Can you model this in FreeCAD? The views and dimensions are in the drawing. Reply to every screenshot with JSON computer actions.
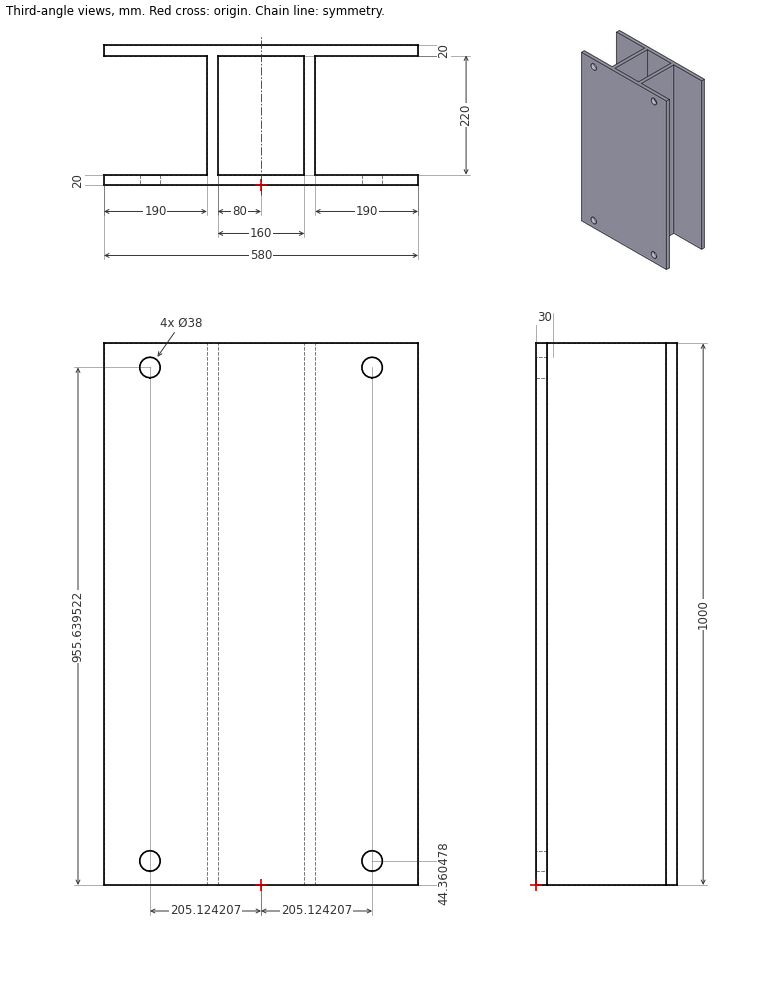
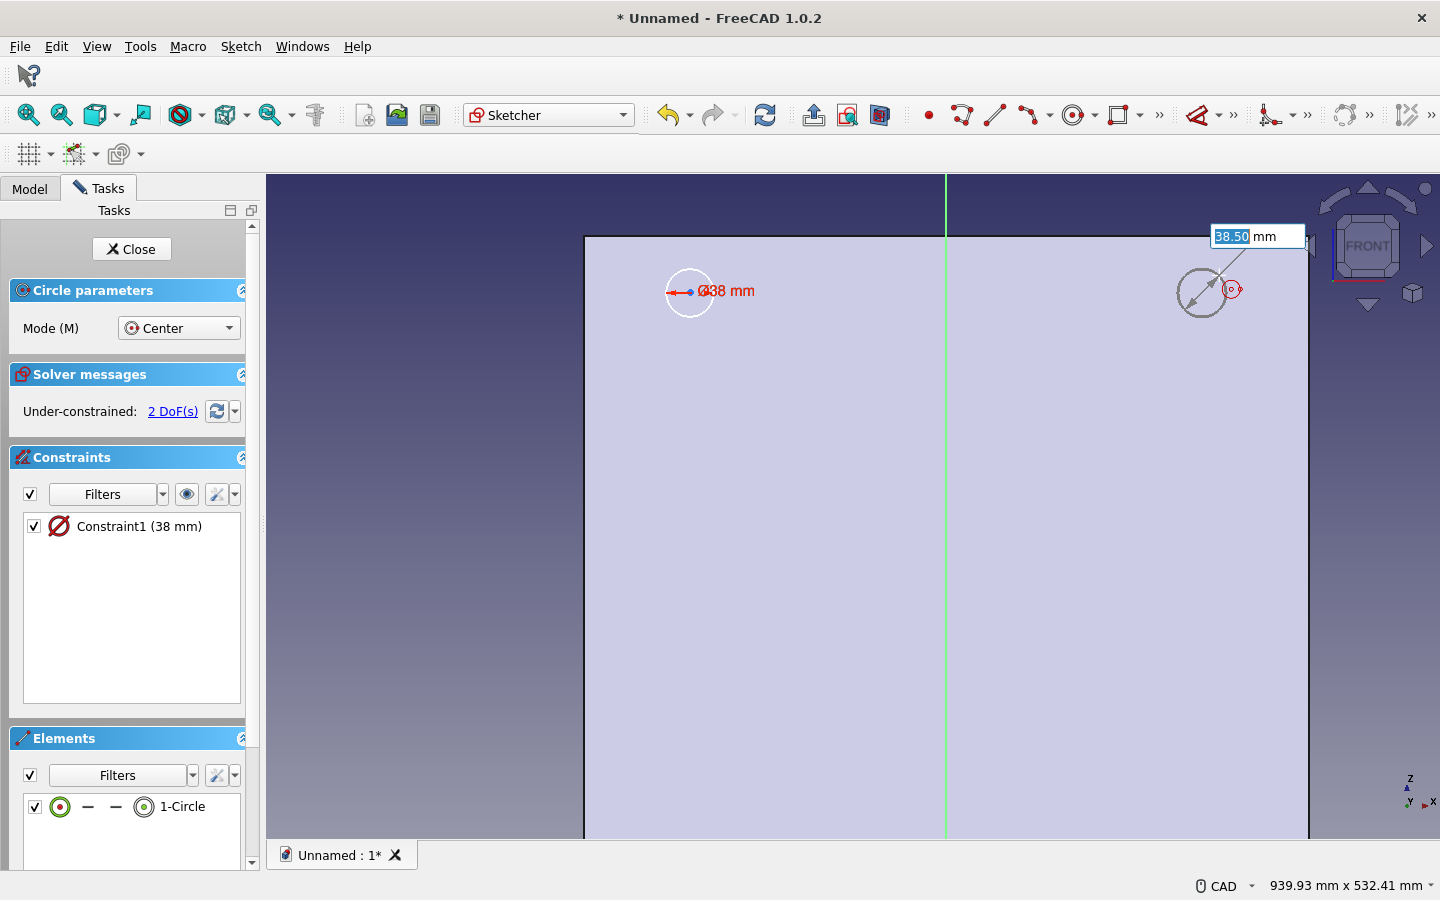
{"action": "type", "text": "38"}
{"action": "key", "text": "Return"}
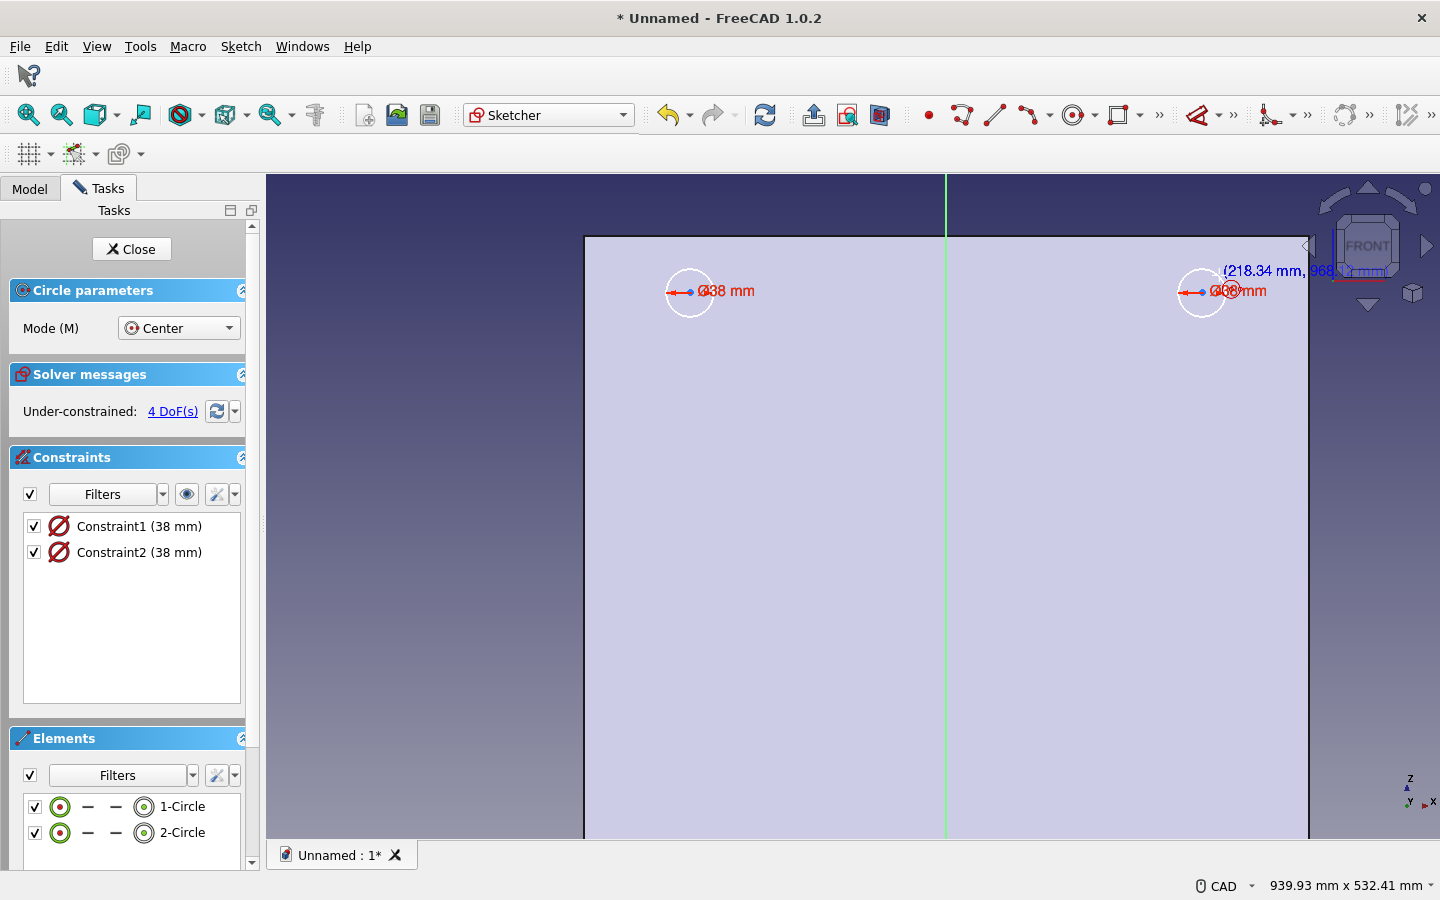
{"action": "scroll", "coordinate": [690, 291], "scroll_direction": "down", "scroll_amount": 5}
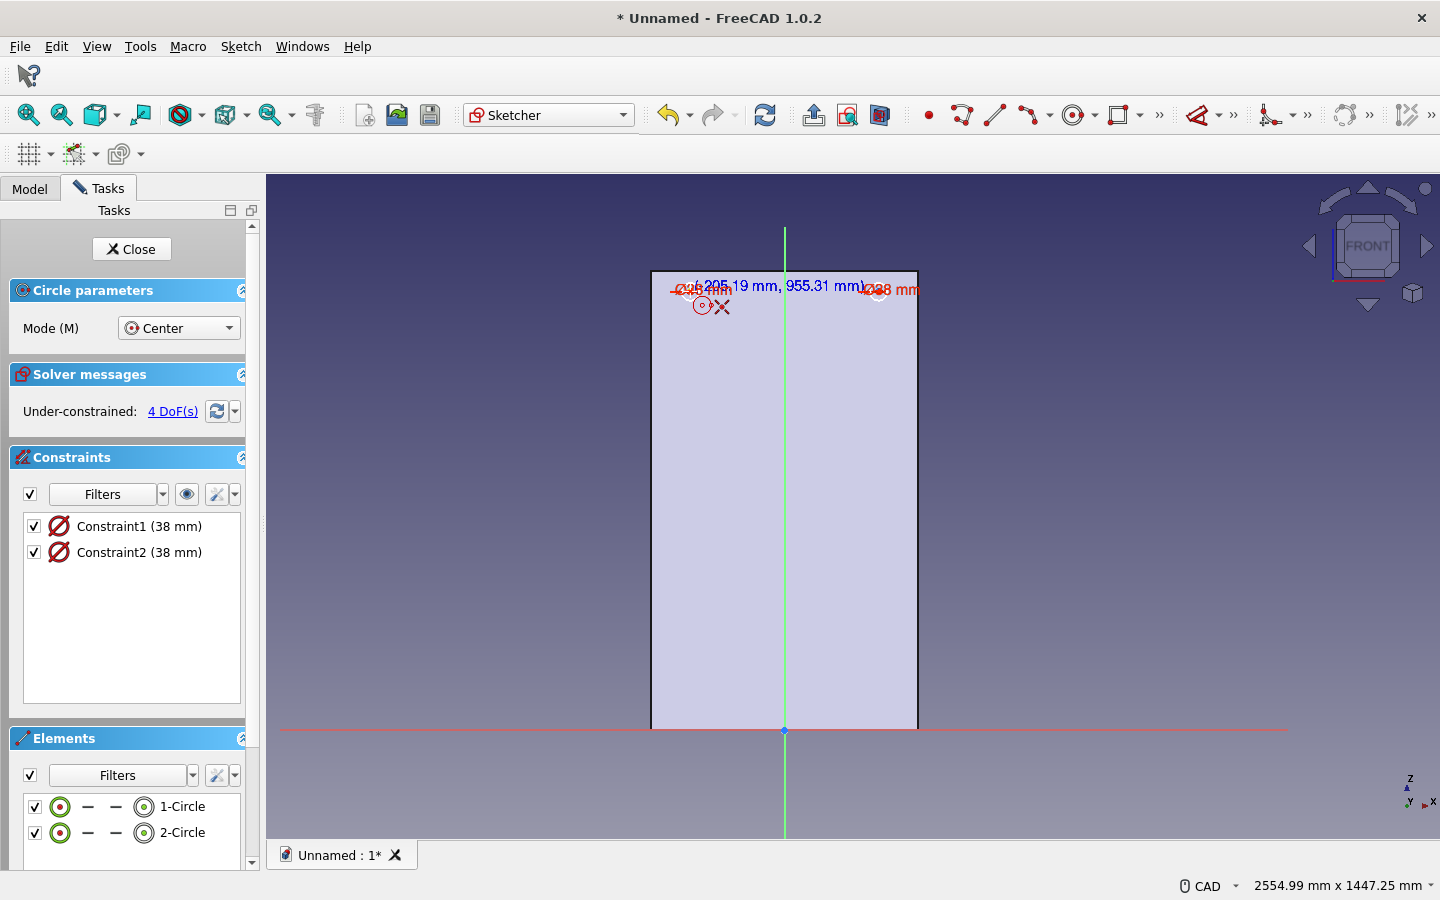
{"action": "scroll", "coordinate": [879, 710], "scroll_direction": "up", "scroll_amount": 5}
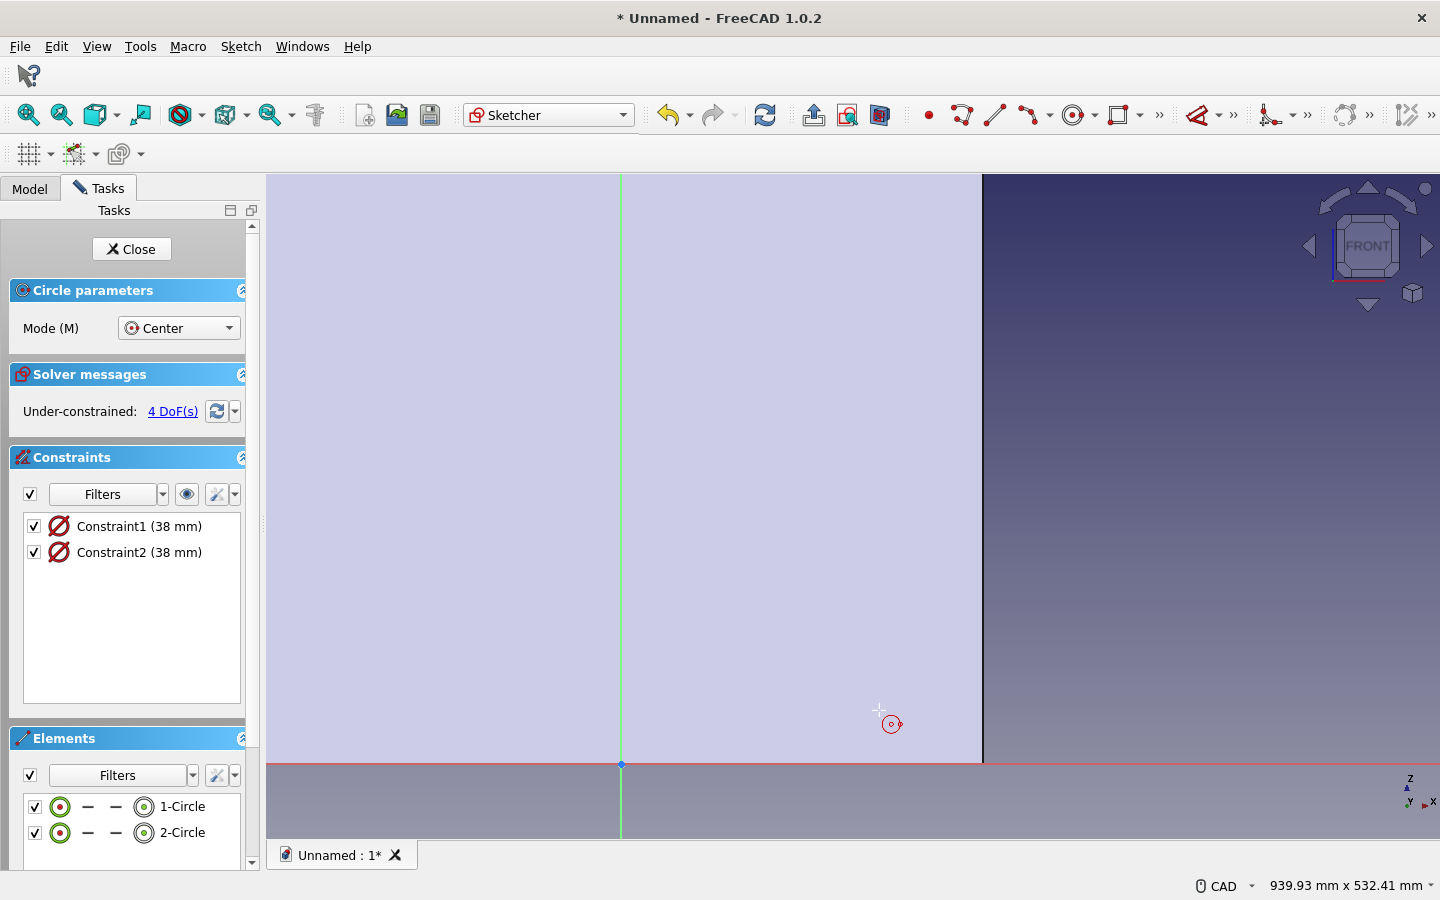
{"action": "left_click", "coordinate": [877, 709]}
{"action": "mouse_move", "coordinate": [894, 692]}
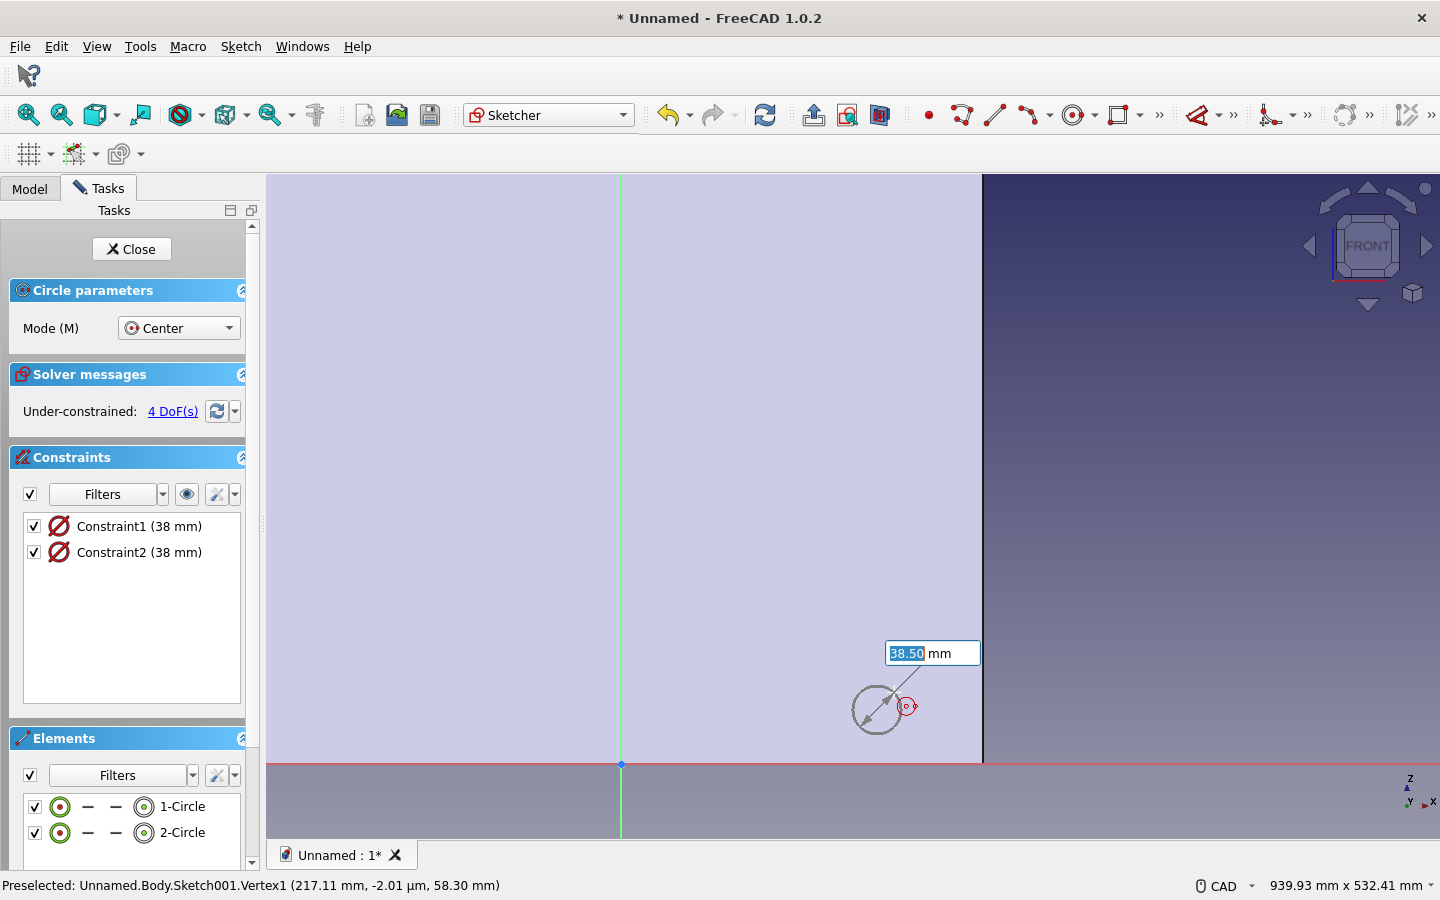
{"action": "type", "text": "38"}
{"action": "key", "text": "Return"}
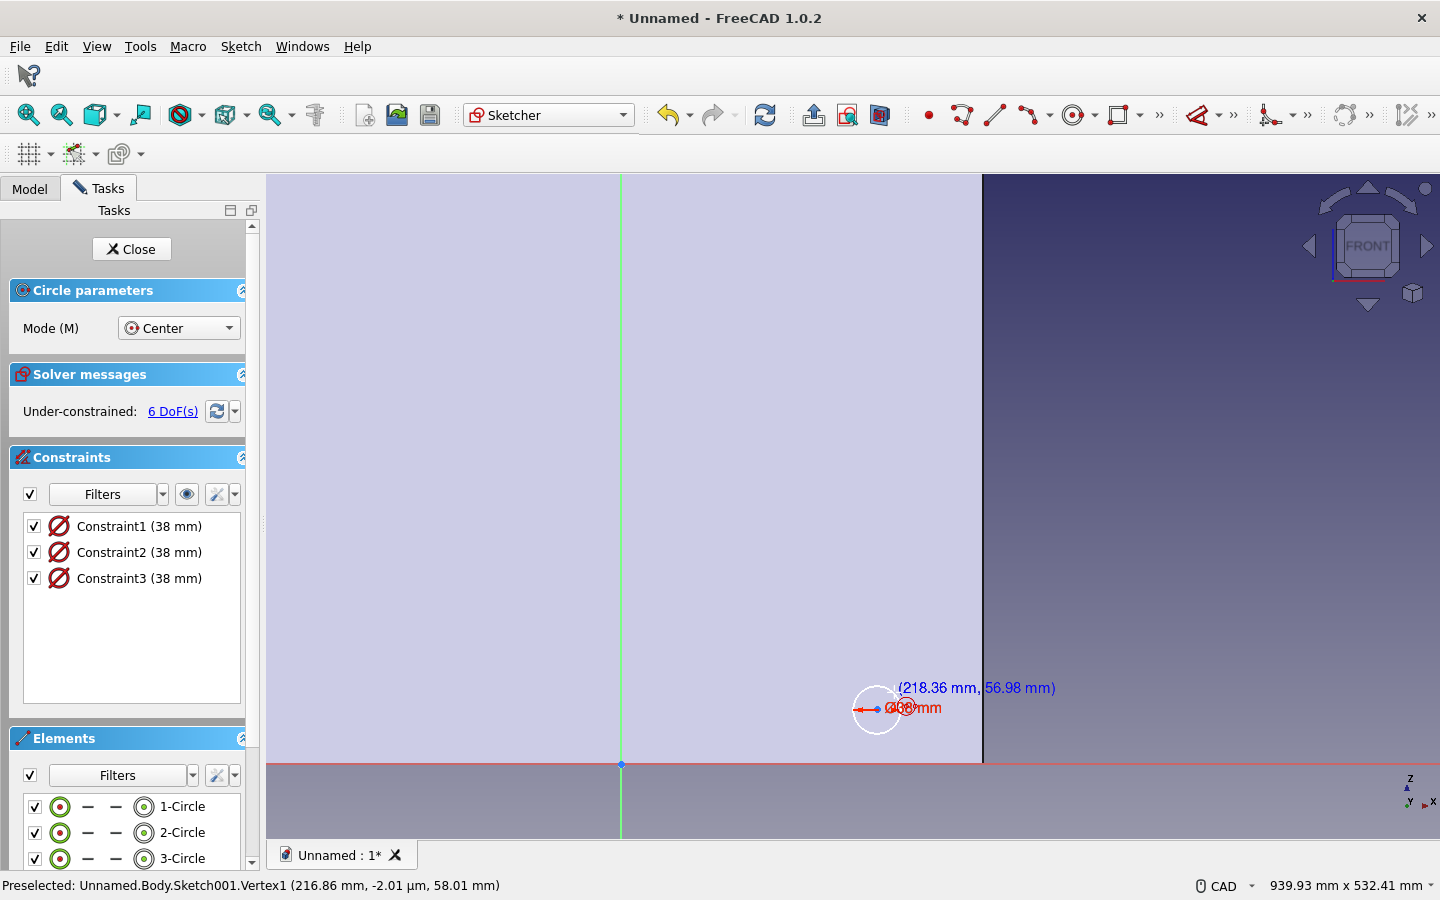
{"action": "left_click", "coordinate": [365, 709]}
{"action": "mouse_move", "coordinate": [382, 692]}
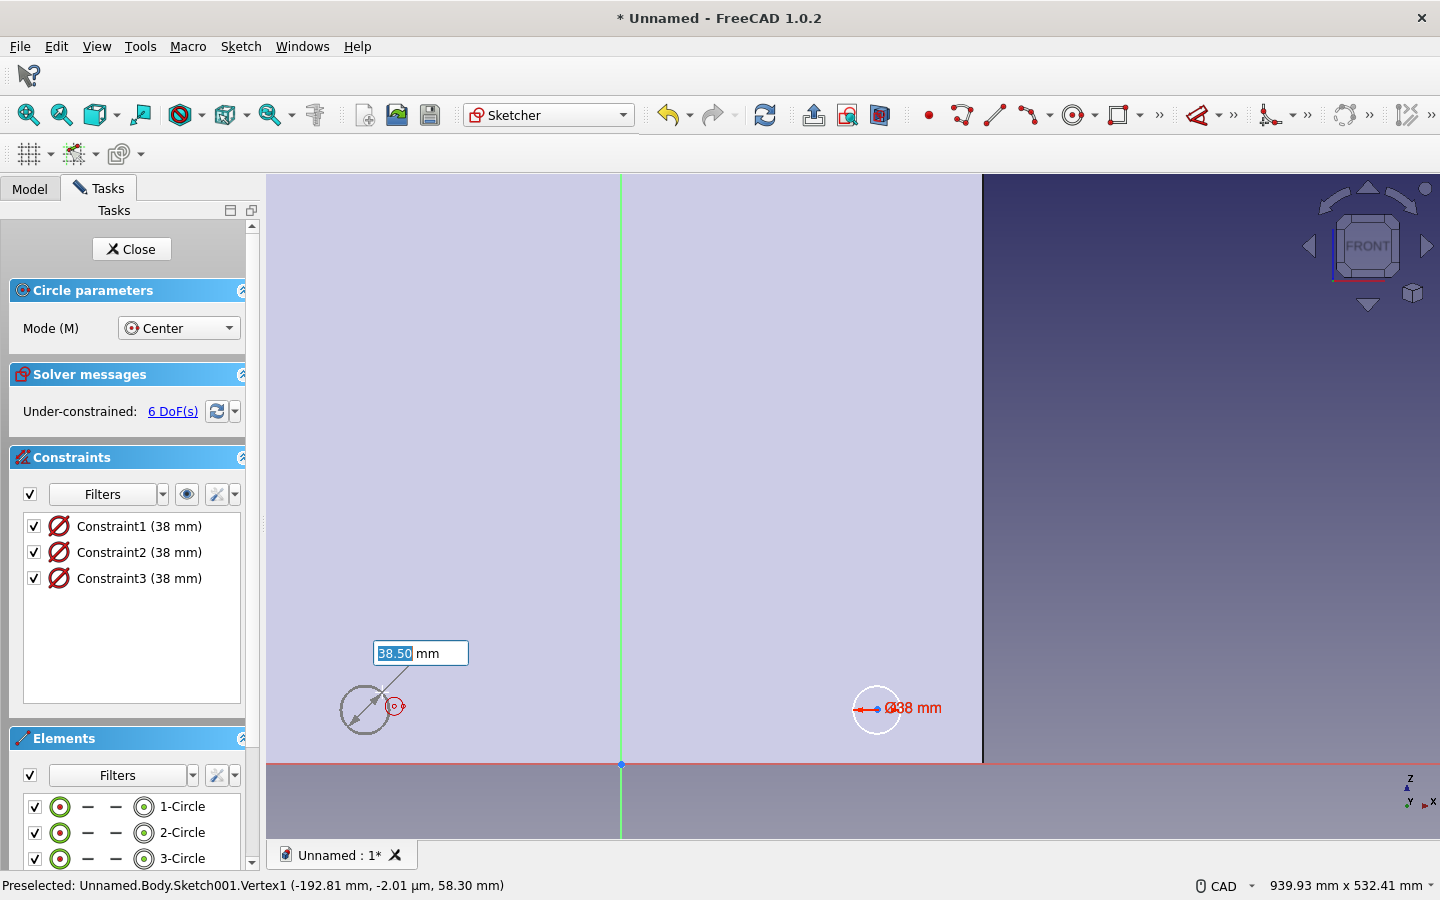
{"action": "type", "text": "38"}
{"action": "key", "text": "Return"}
{"action": "key", "text": "Escape"}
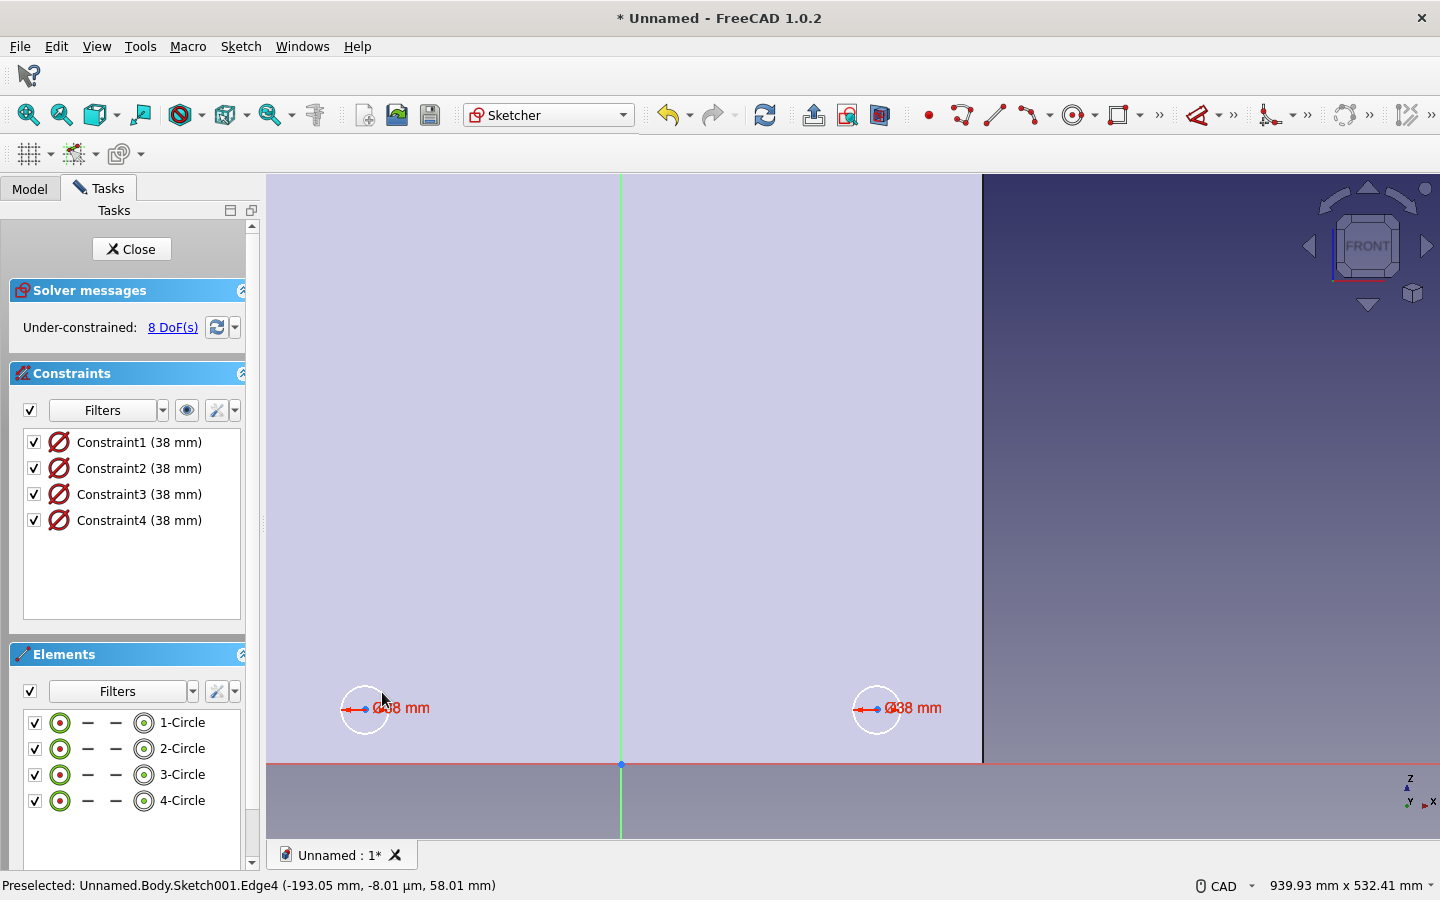
{"action": "scroll", "coordinate": [880, 711], "scroll_direction": "down", "scroll_amount": 5}